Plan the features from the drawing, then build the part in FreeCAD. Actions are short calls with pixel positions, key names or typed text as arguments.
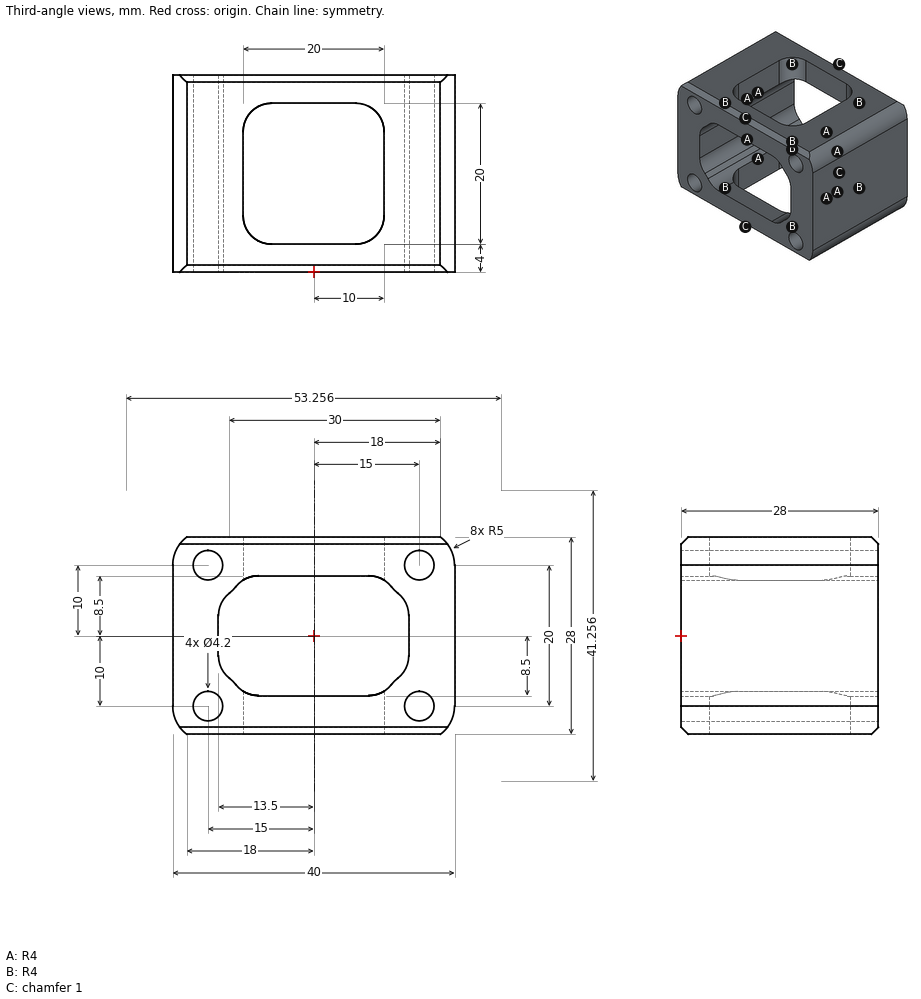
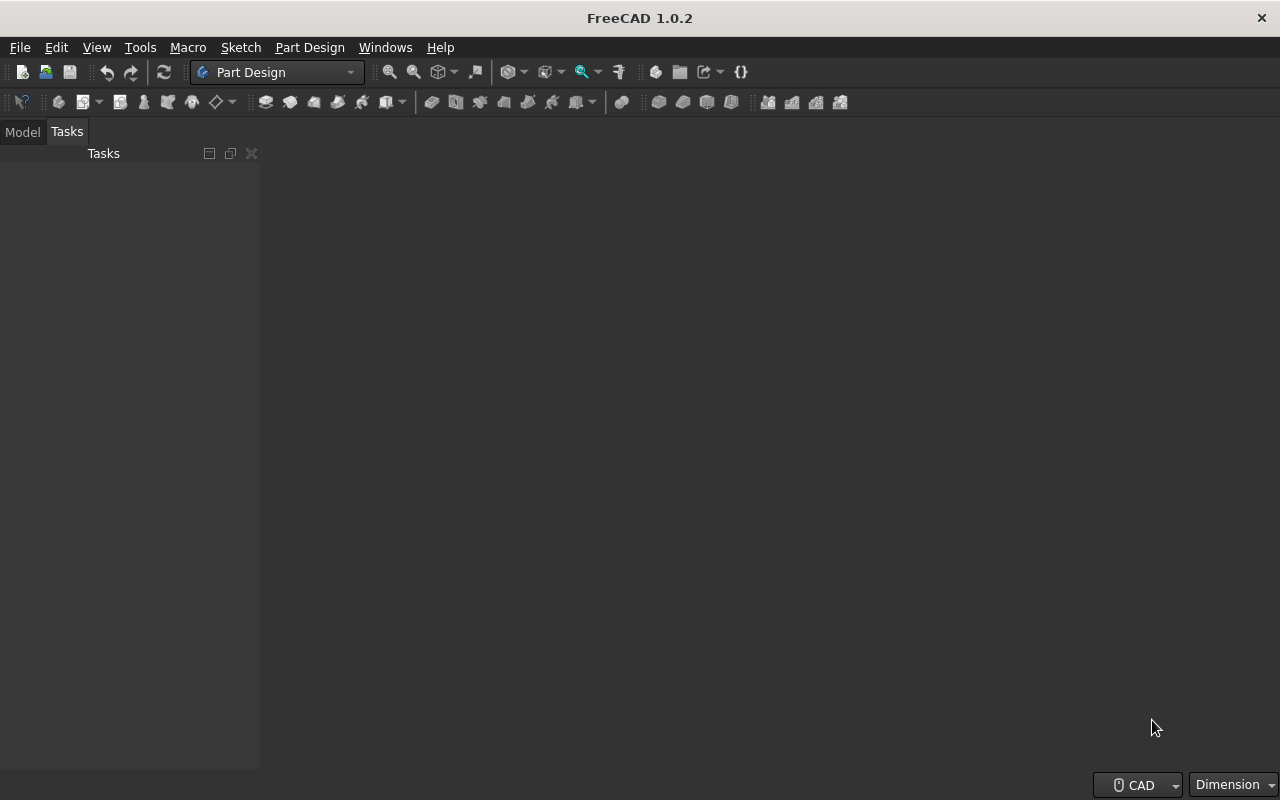
click(984, 72)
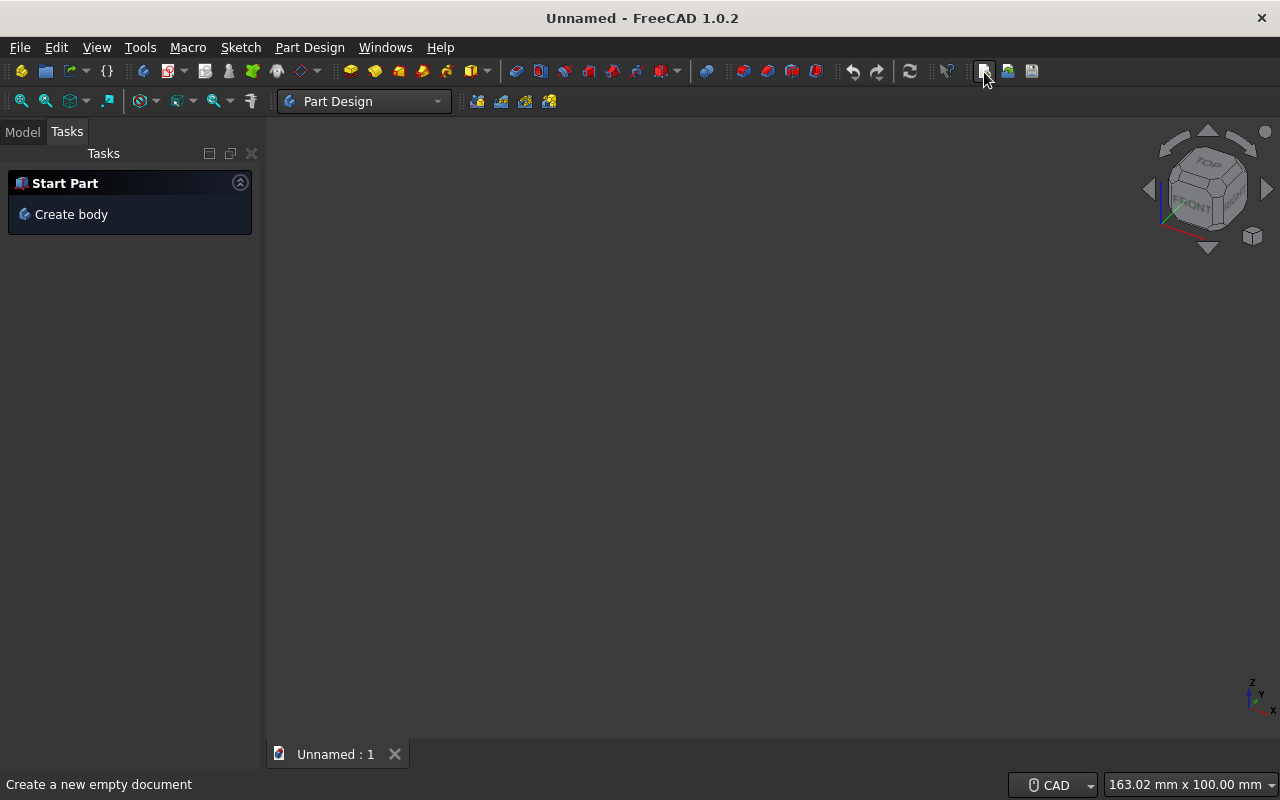
click(168, 72)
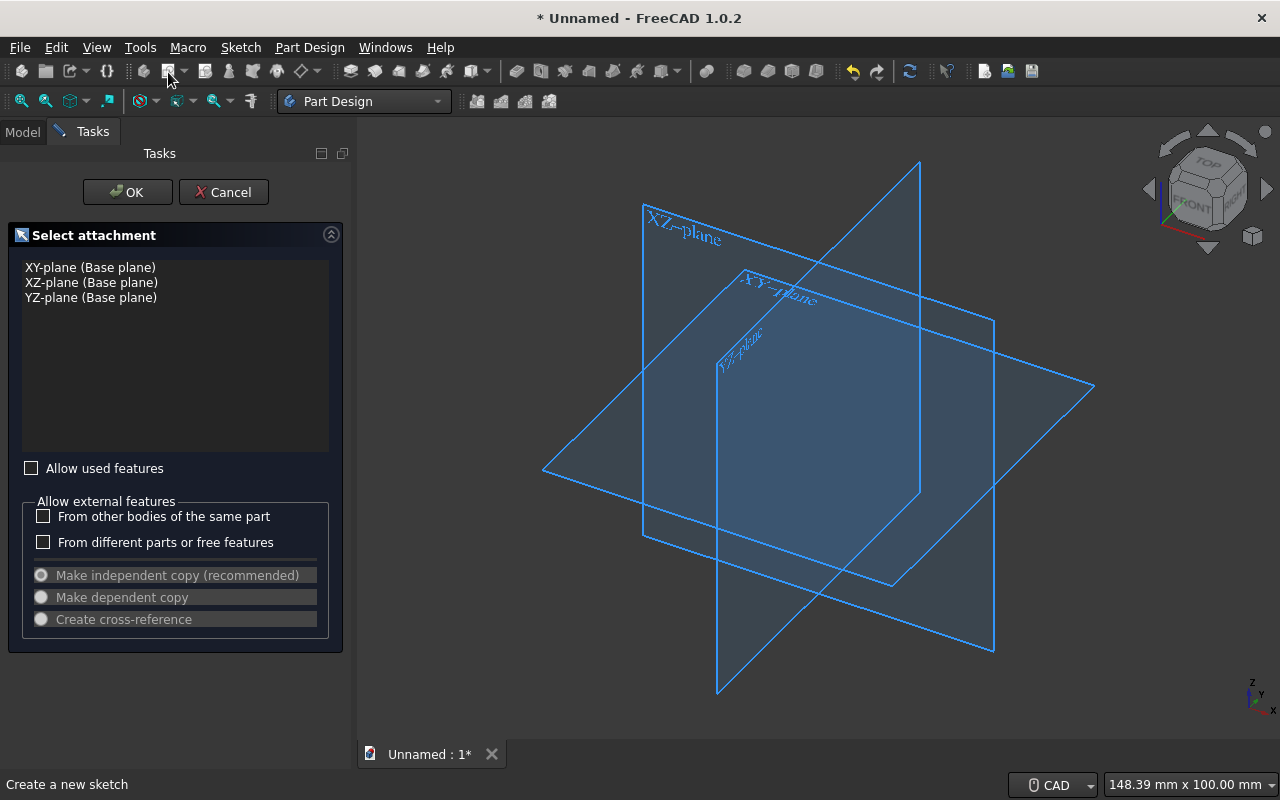
click(82, 282)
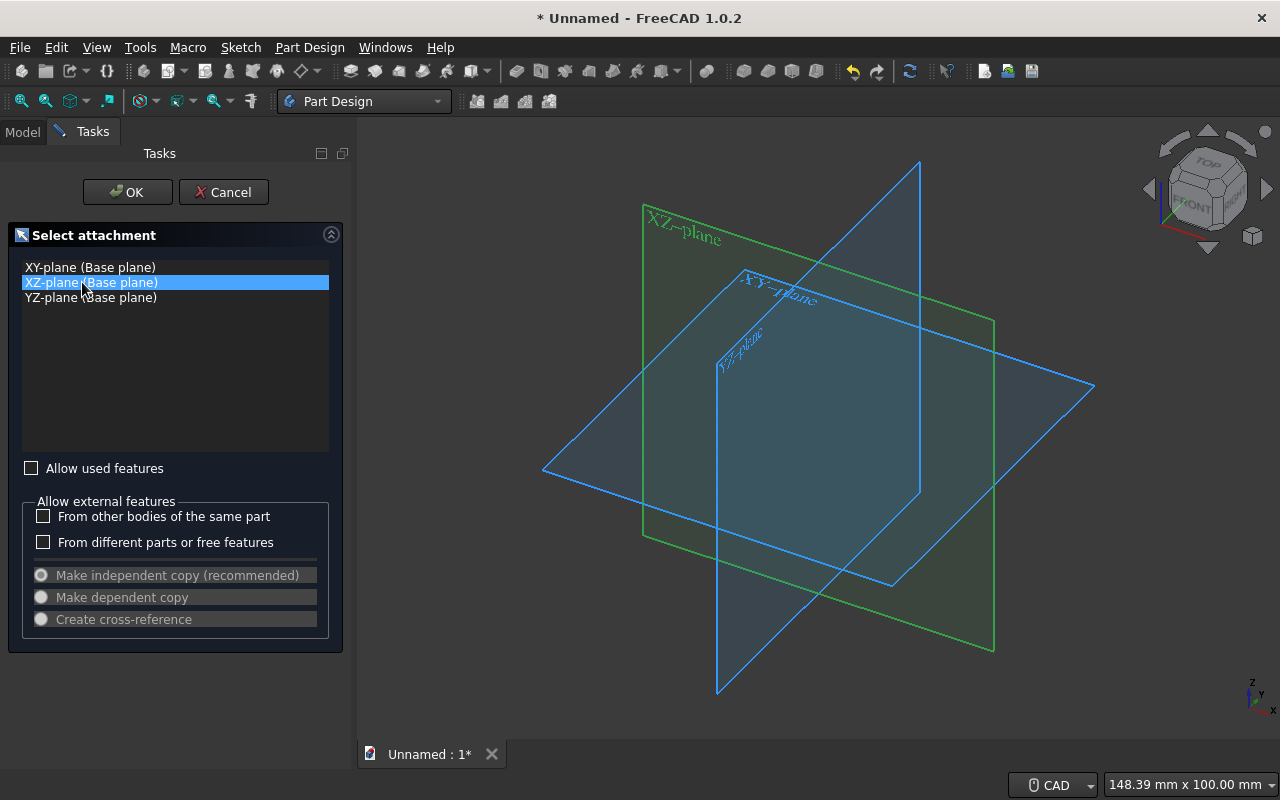
click(128, 192)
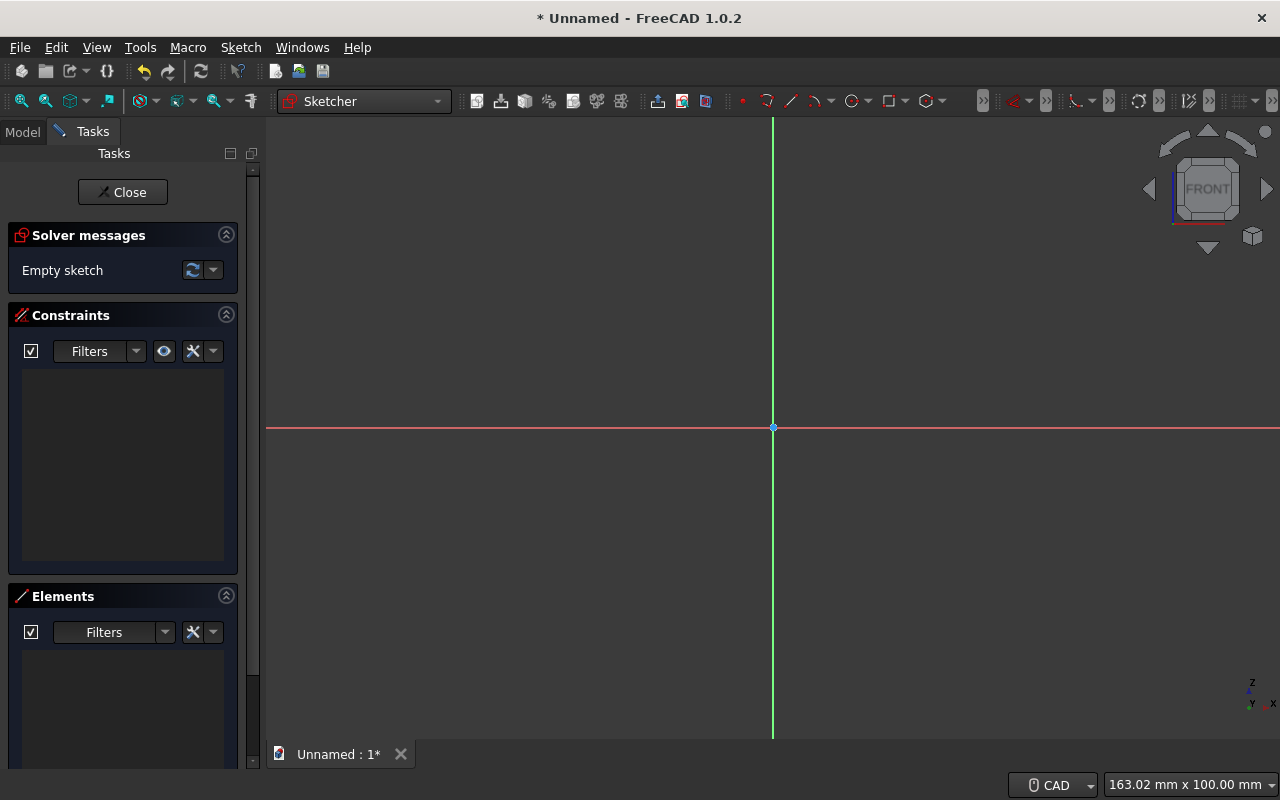
scroll(829, 428, up, 4)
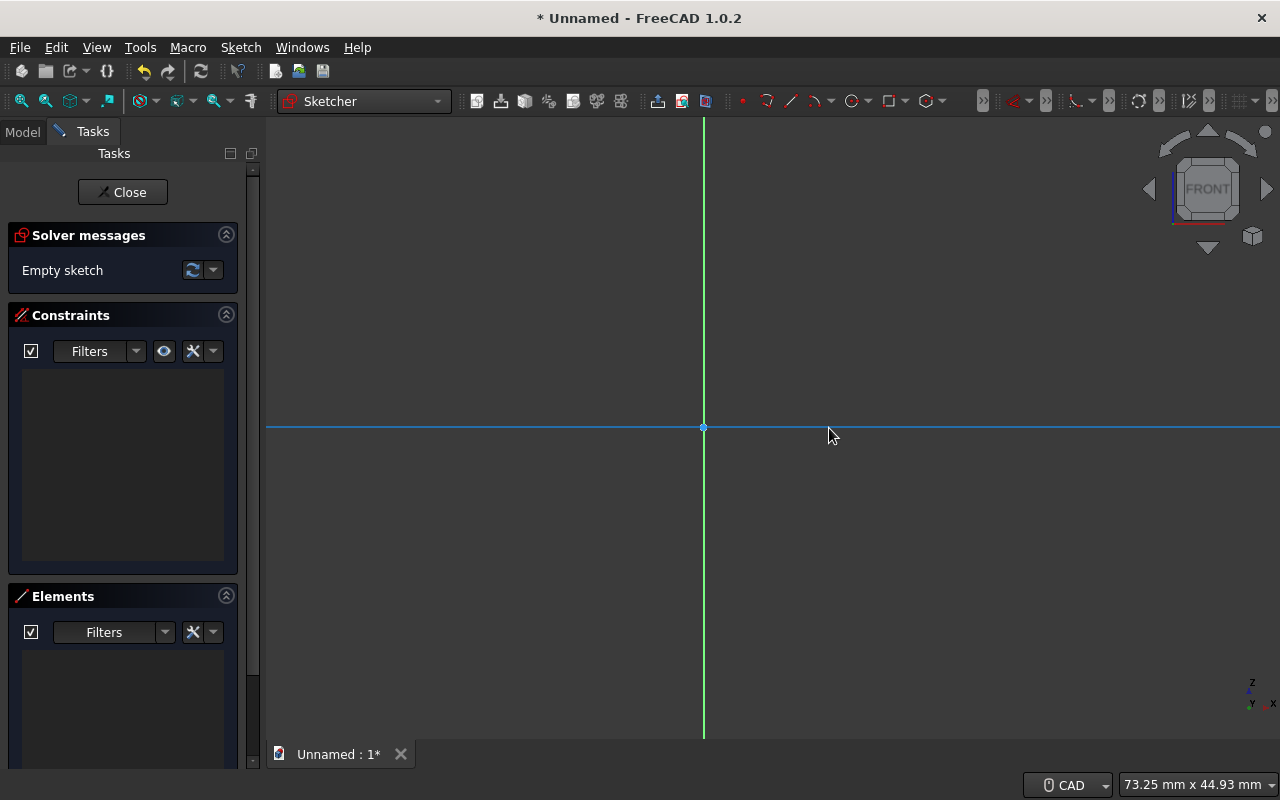
key(g)
key(v)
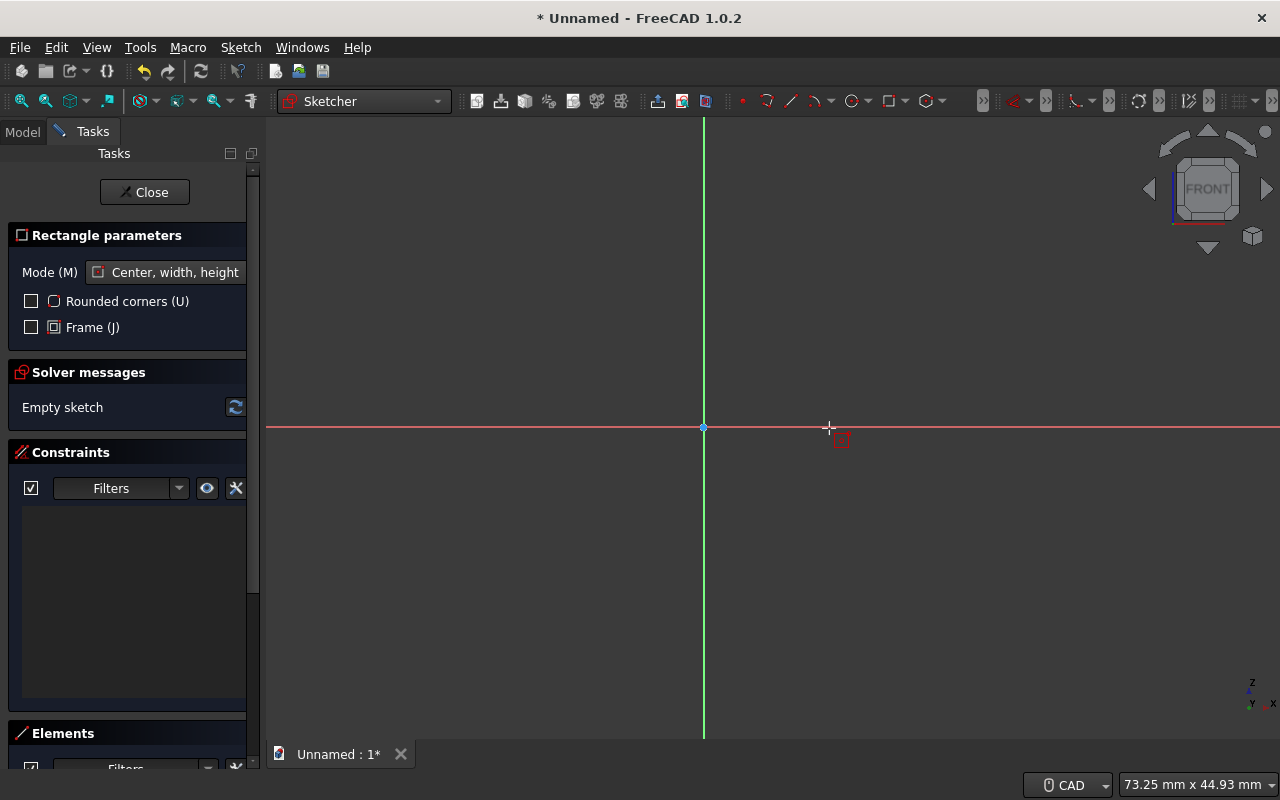
click(704, 427)
click(981, 234)
key(Escape)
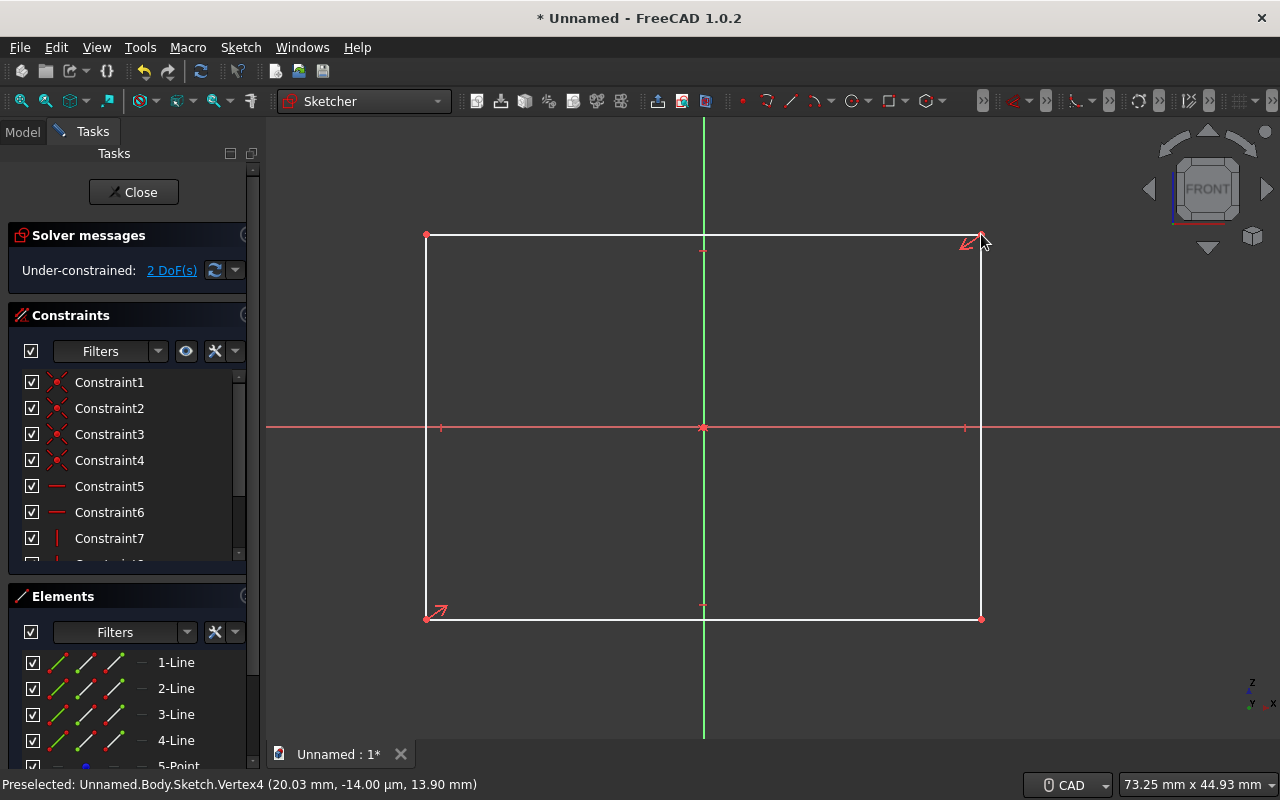
click(593, 620)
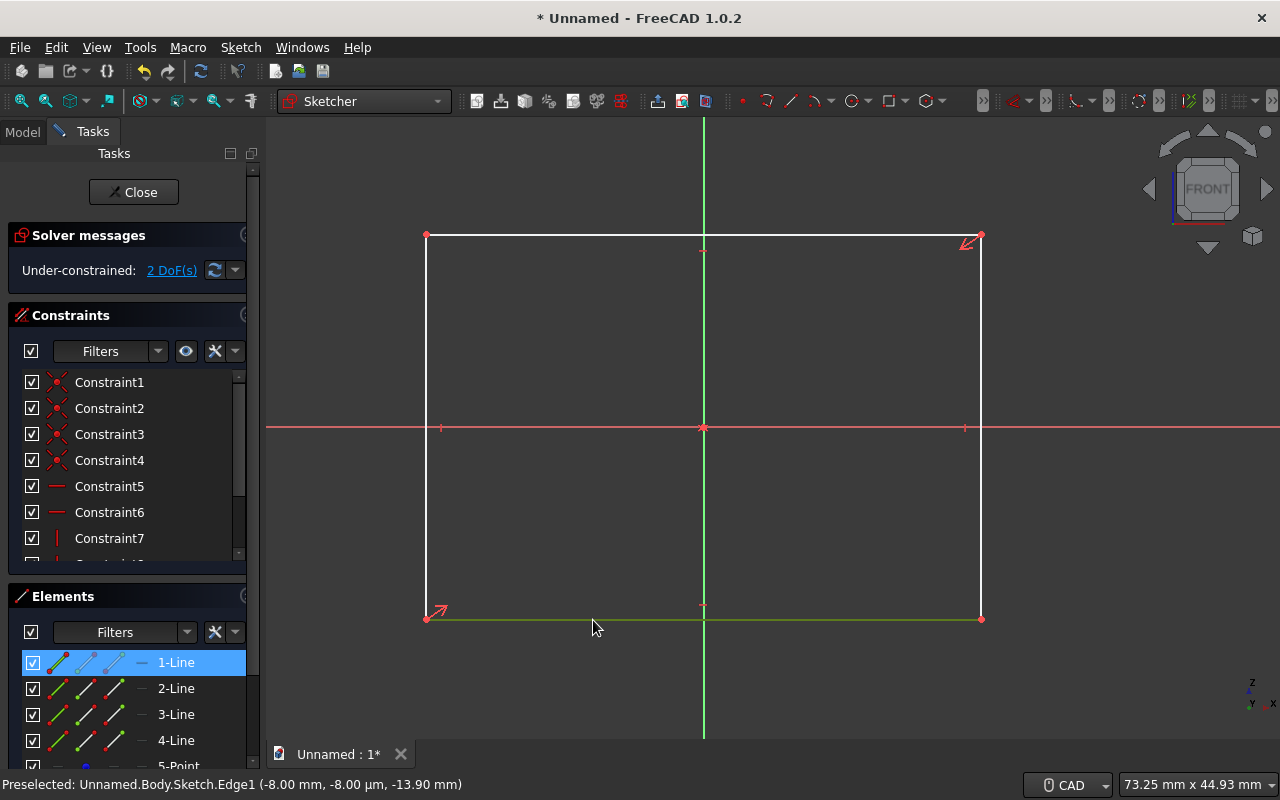
key(l)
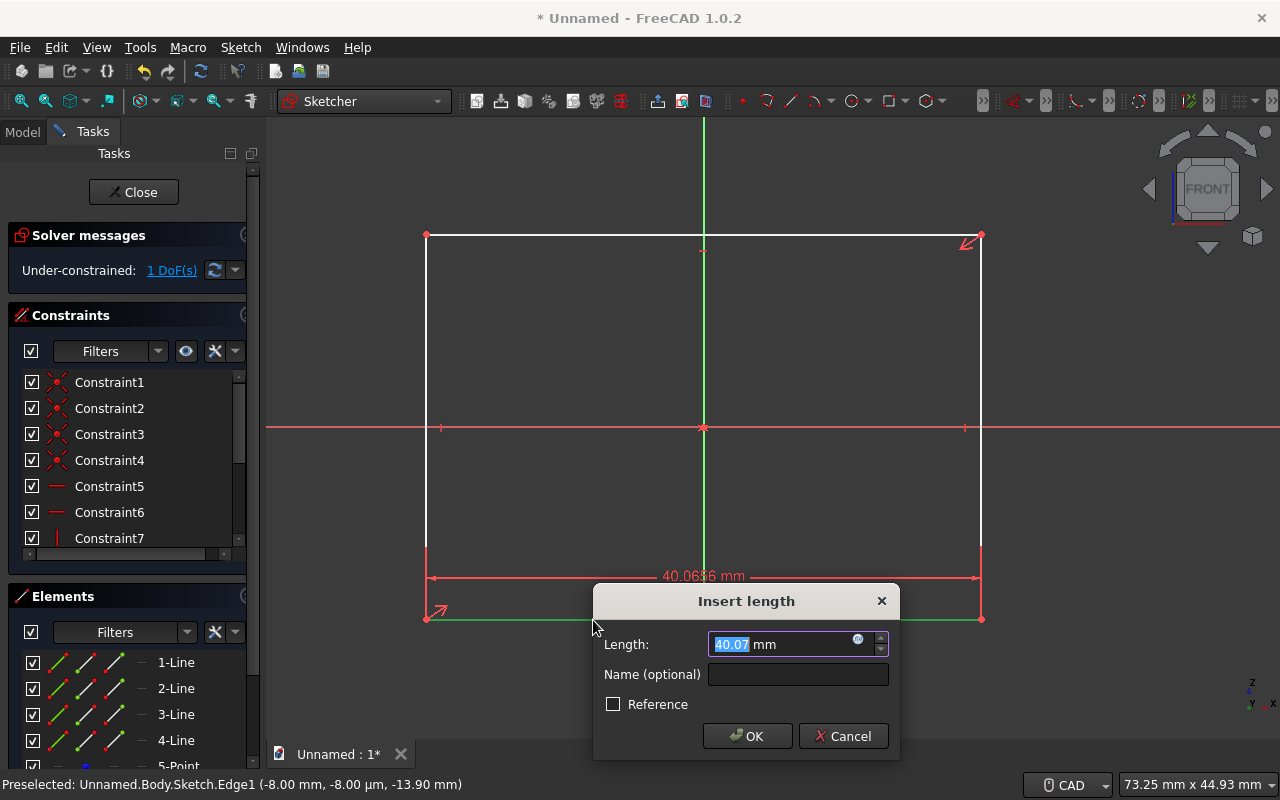
text(40)
key(Return)